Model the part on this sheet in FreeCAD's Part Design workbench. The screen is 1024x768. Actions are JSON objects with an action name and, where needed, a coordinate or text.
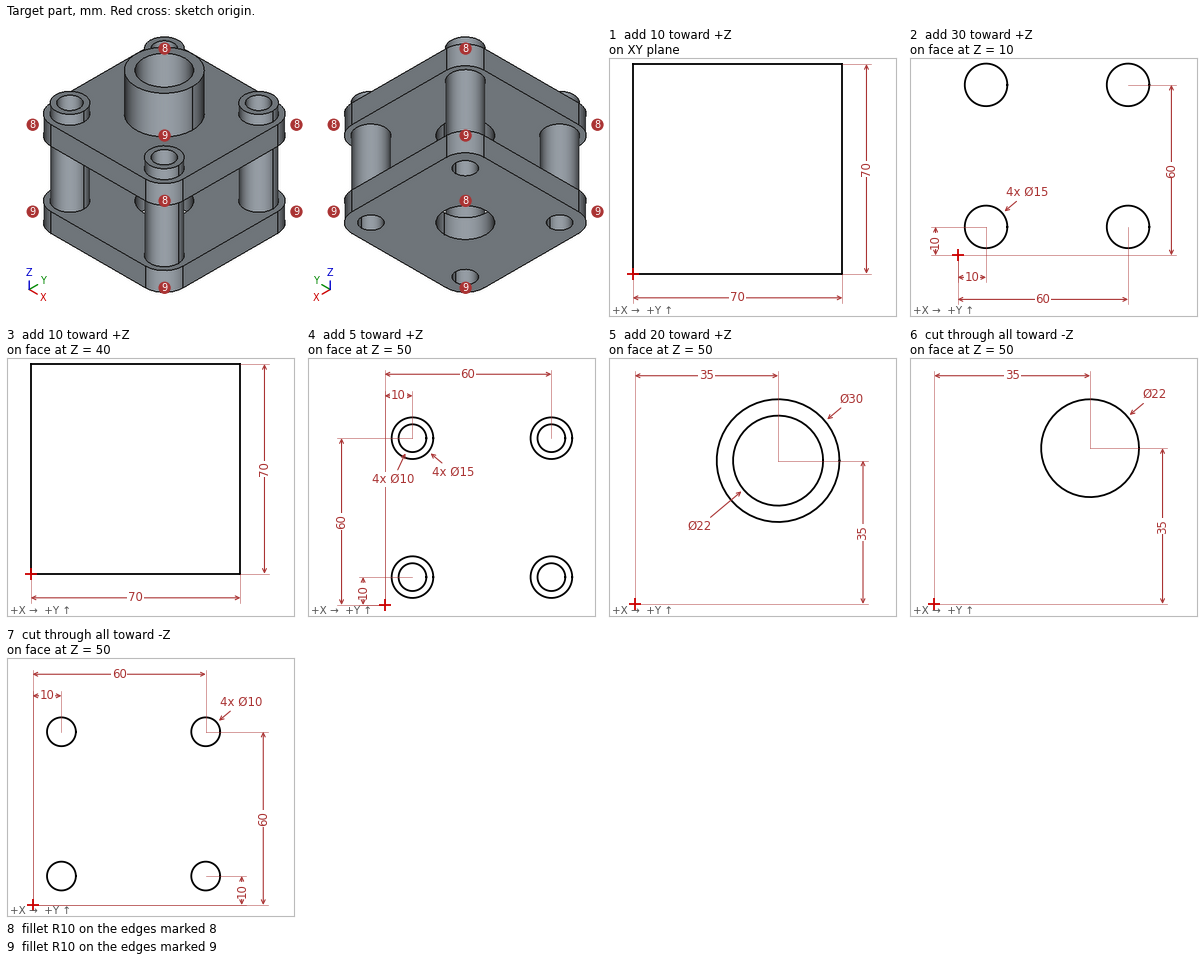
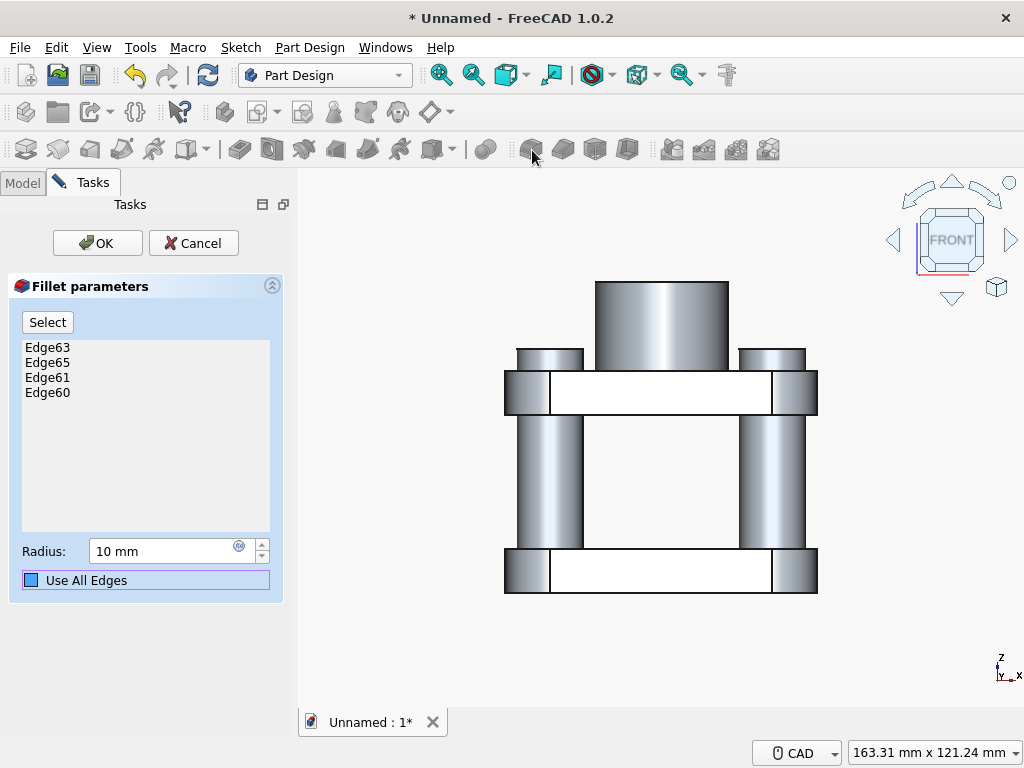
{"action": "left_click", "coordinate": [98, 243]}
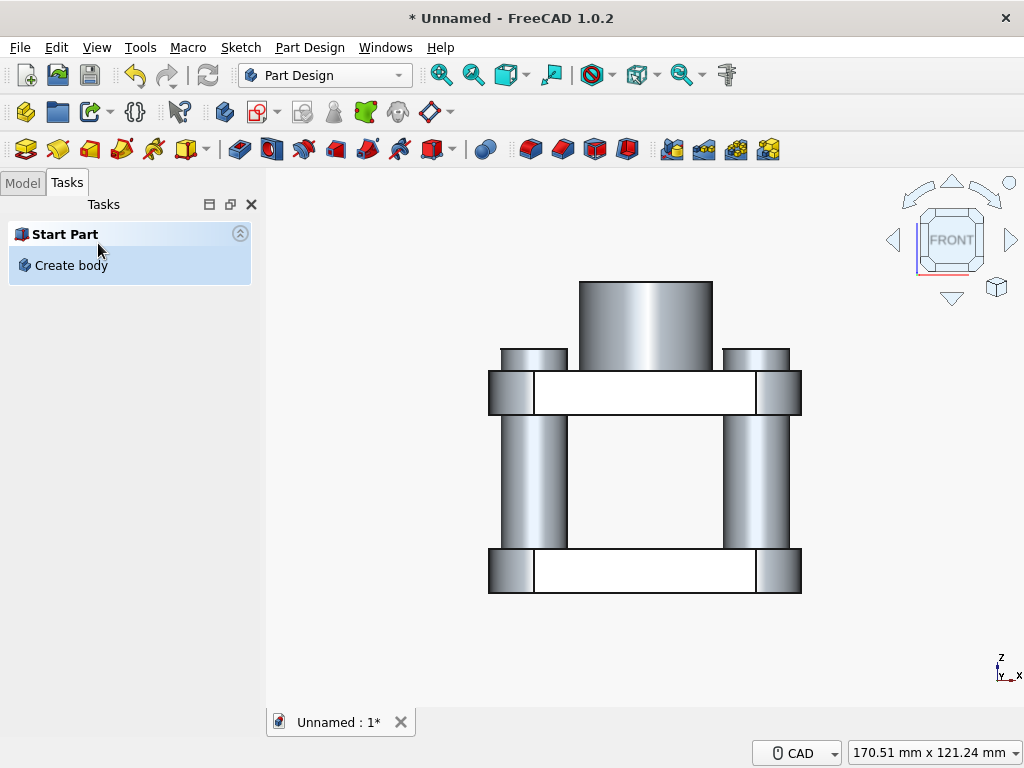
{"action": "key", "text": "0"}